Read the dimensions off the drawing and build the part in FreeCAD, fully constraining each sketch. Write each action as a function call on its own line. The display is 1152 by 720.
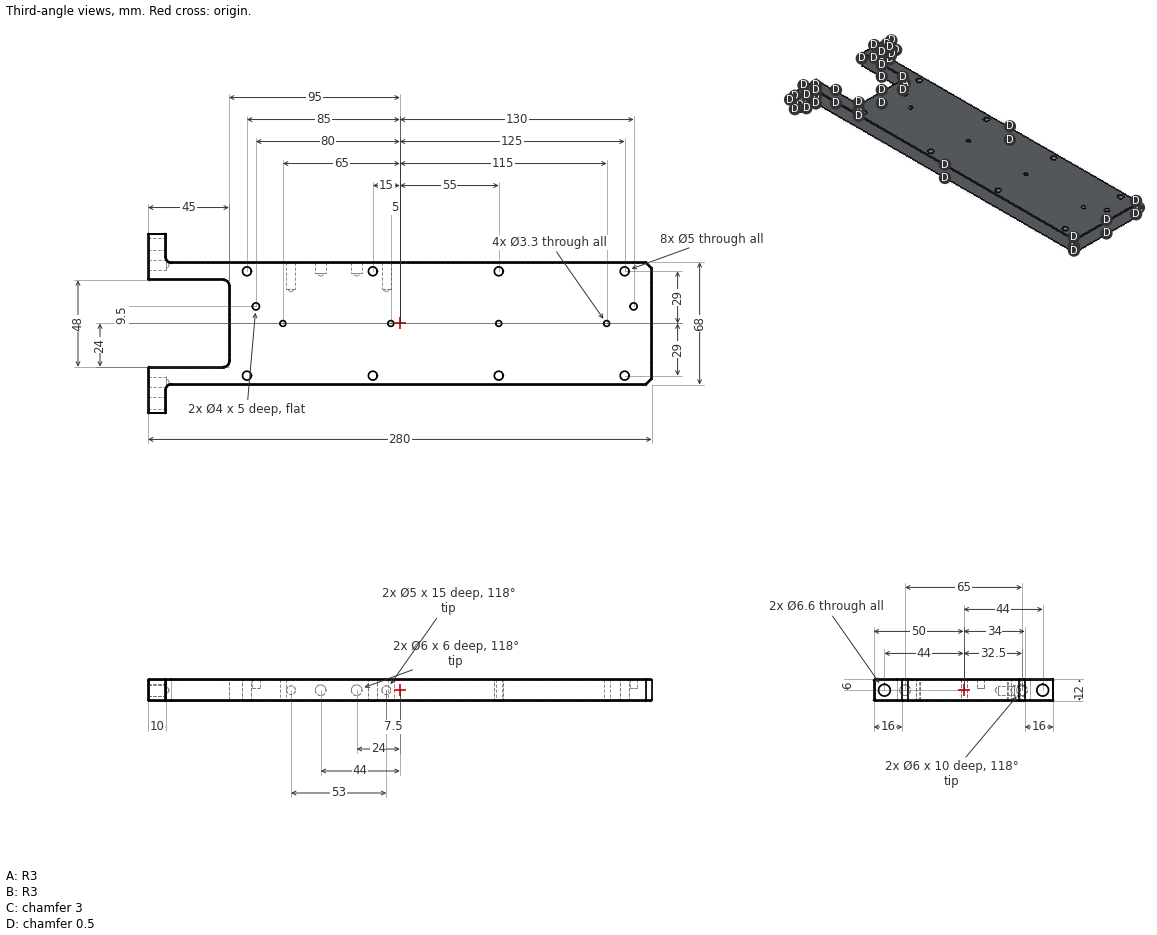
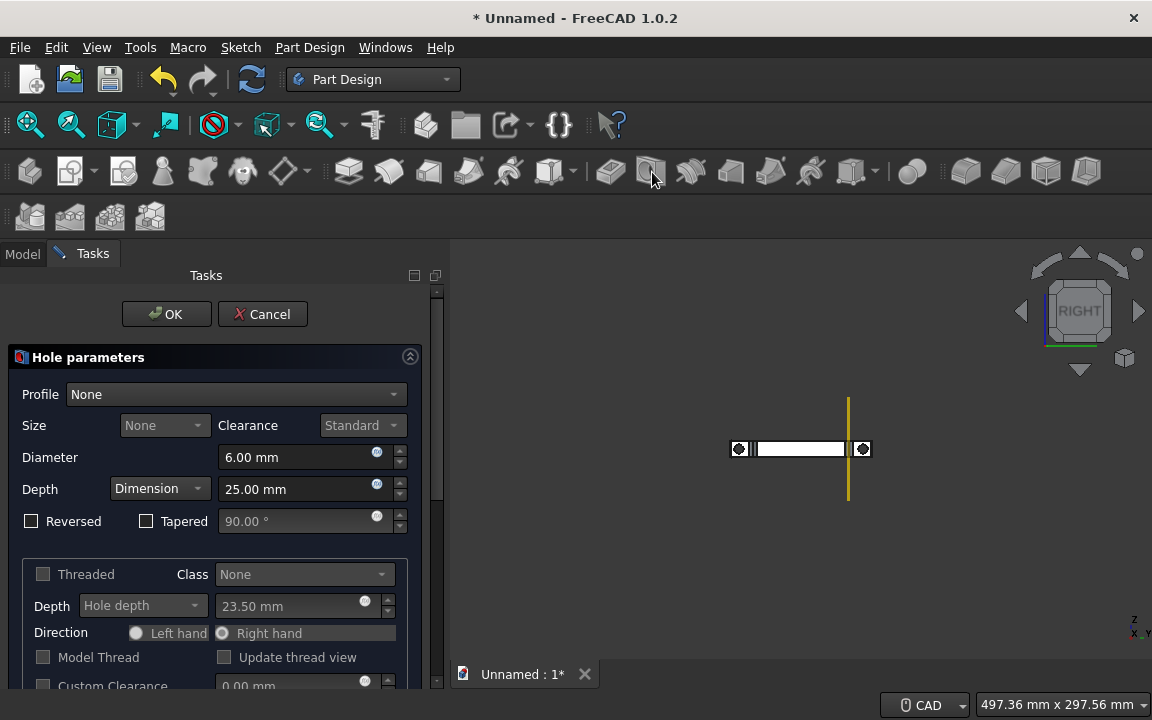
triple_click(305, 457)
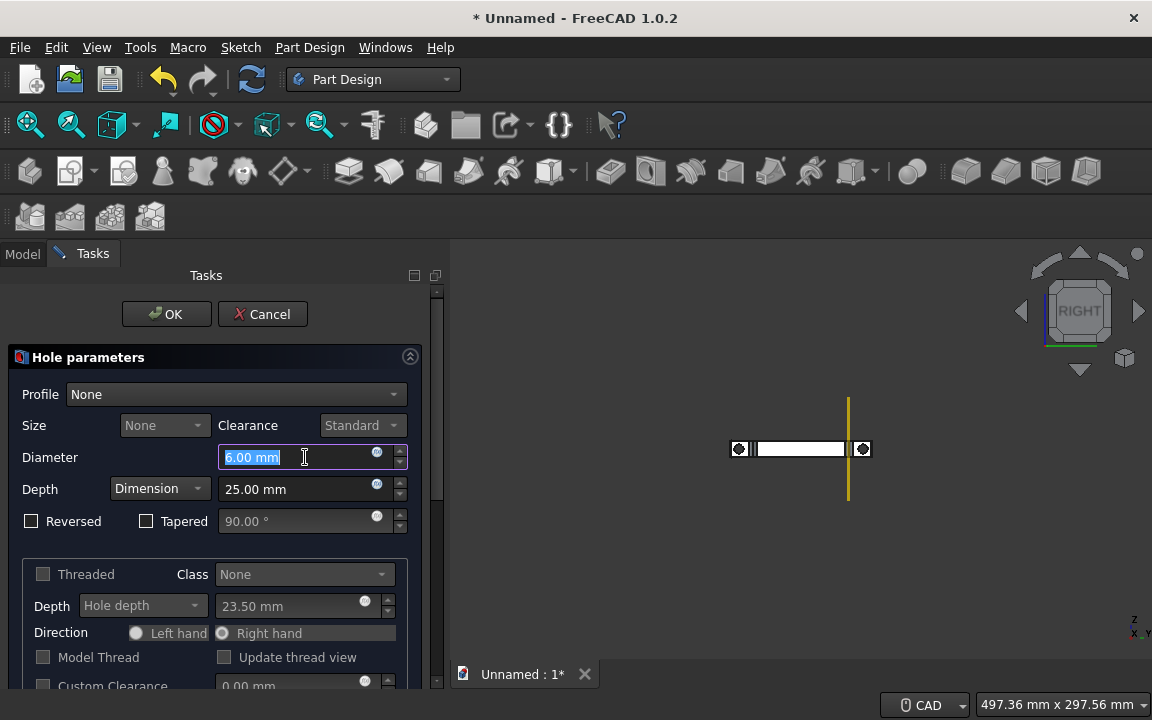
text(5)
key(Tab)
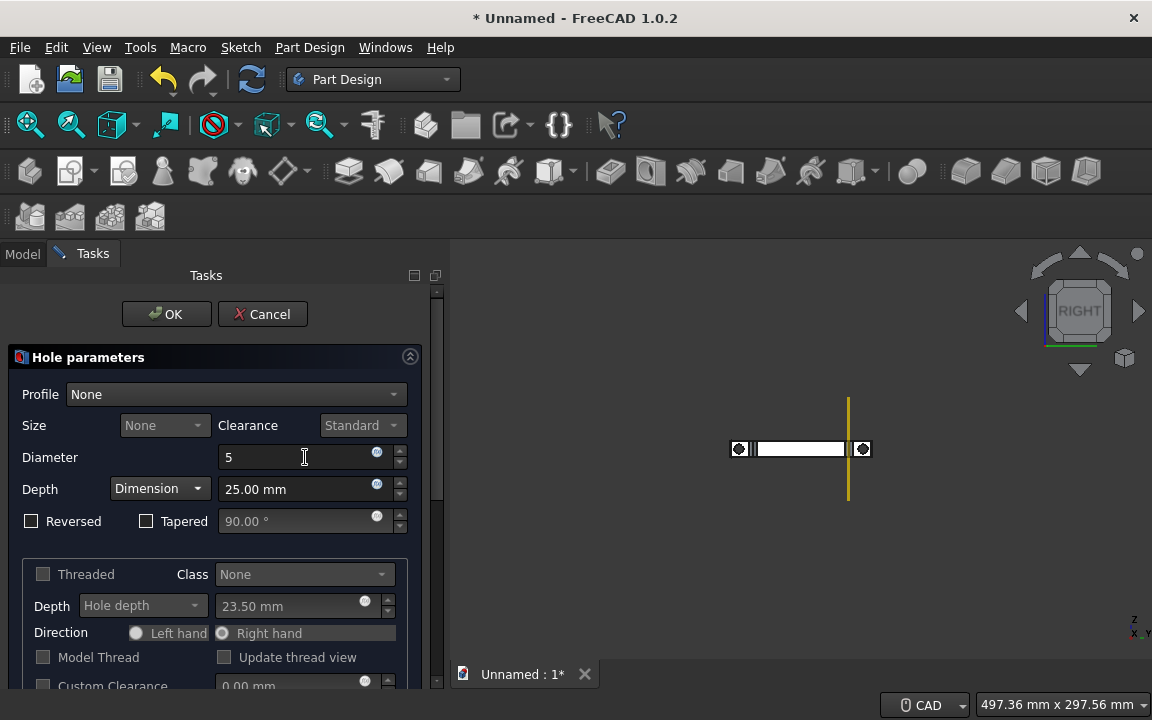
triple_click(305, 489)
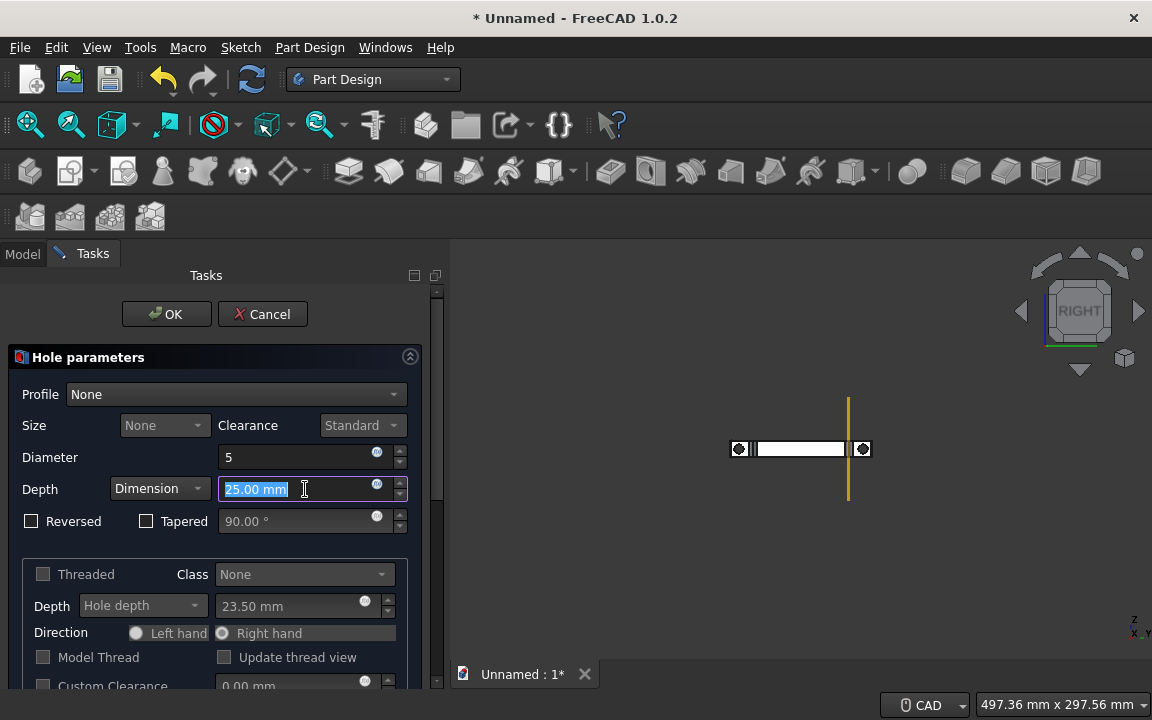
text(15)
key(Tab)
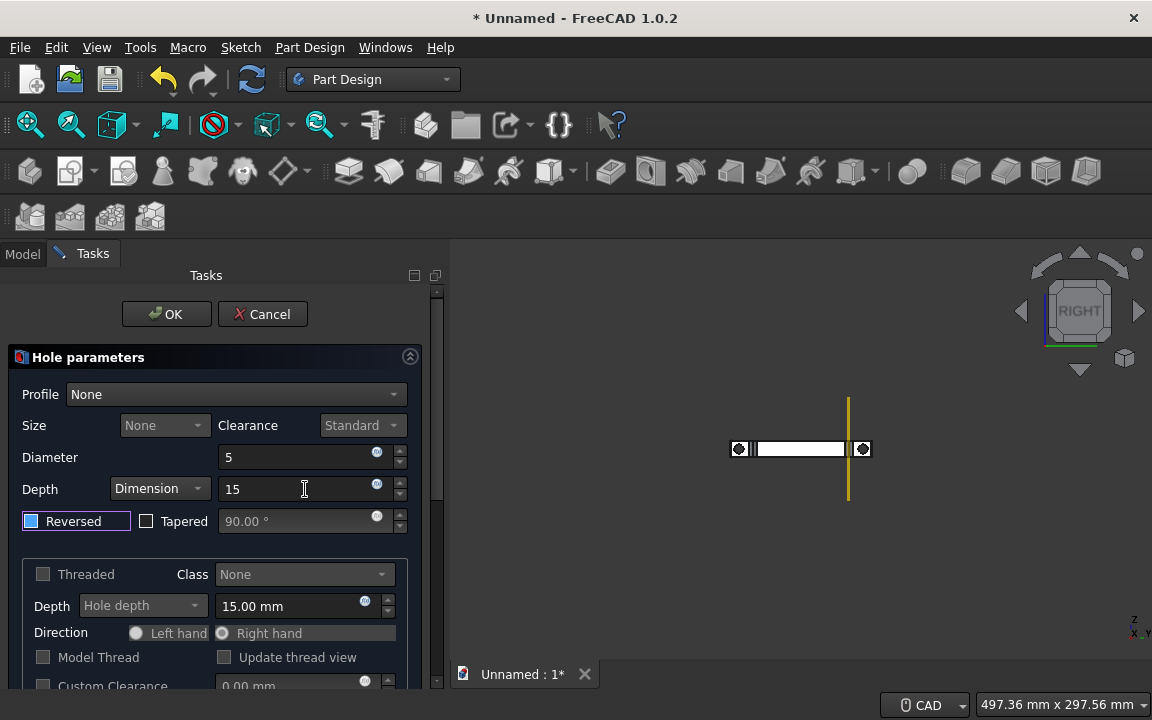
click(30, 521)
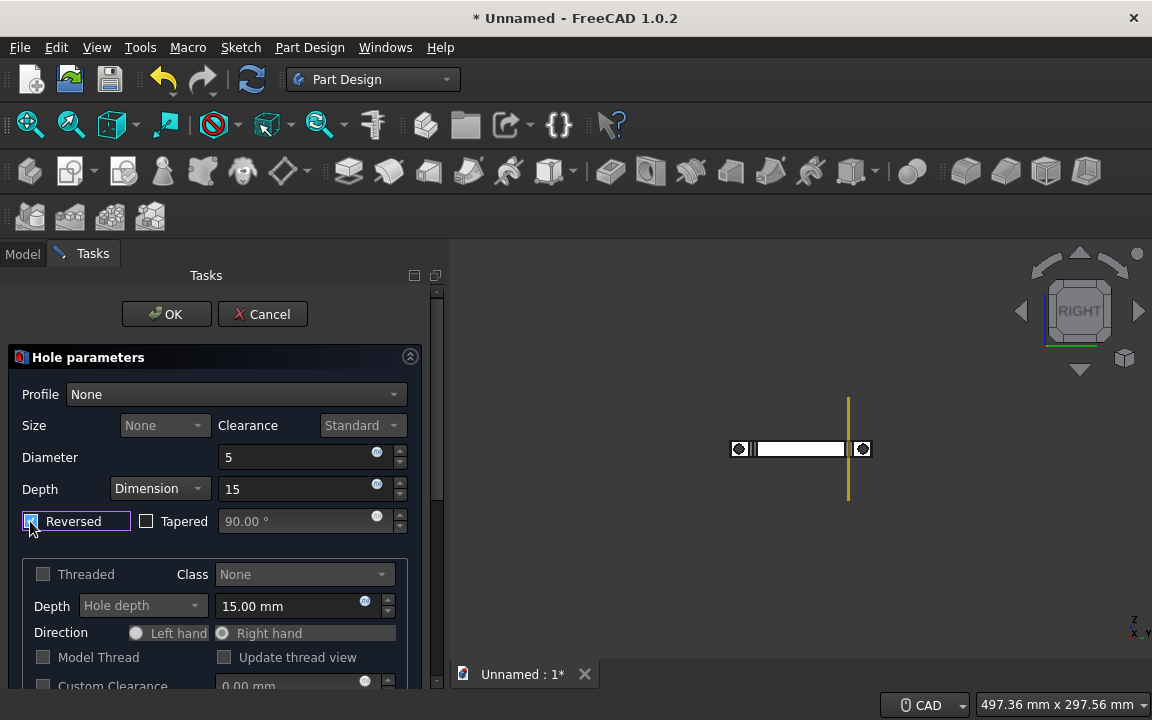
click(167, 314)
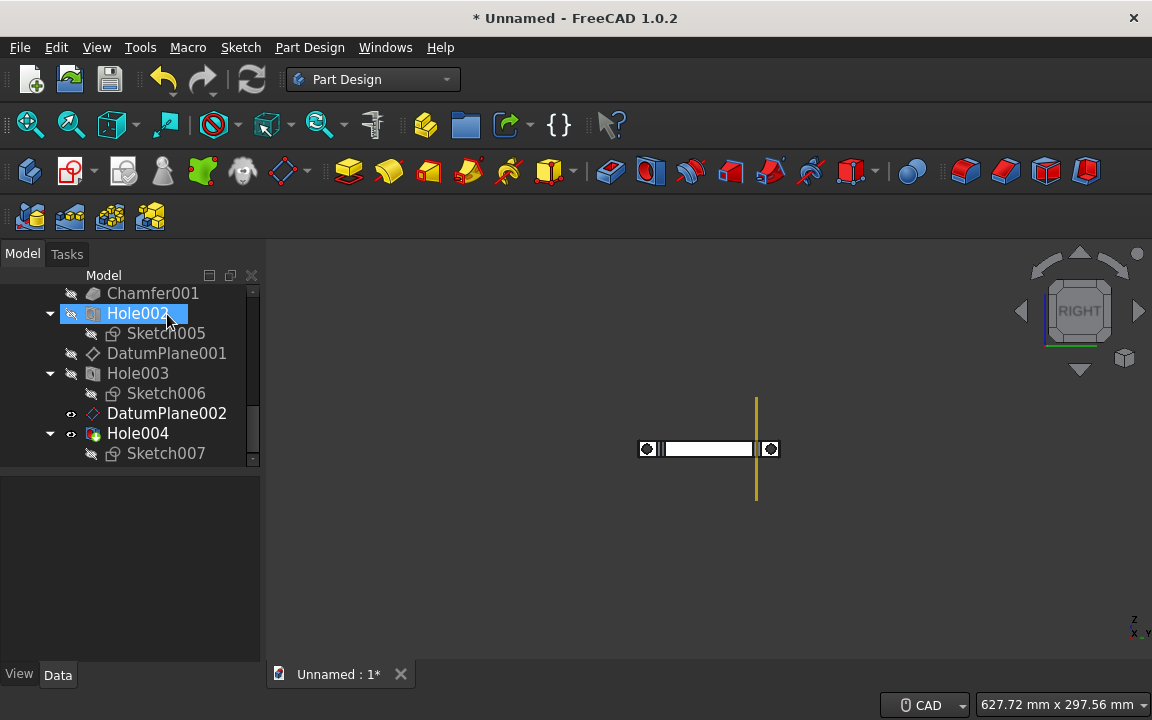
click(116, 414)
key(space)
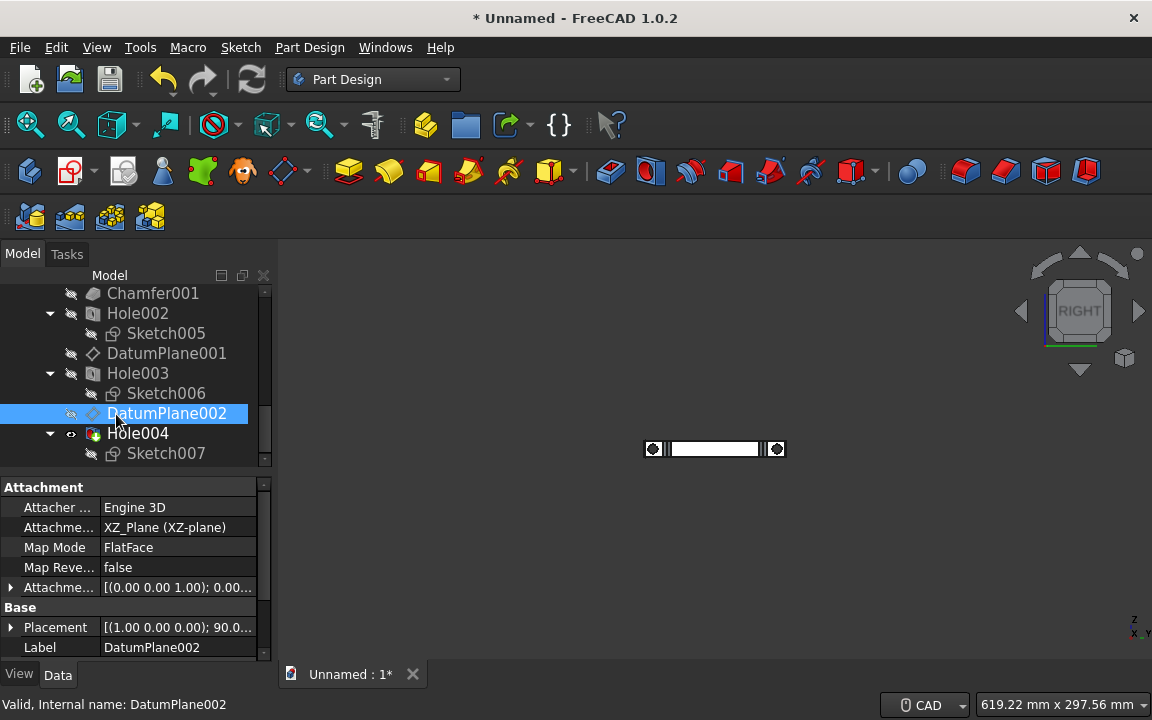
key(v)
key(f)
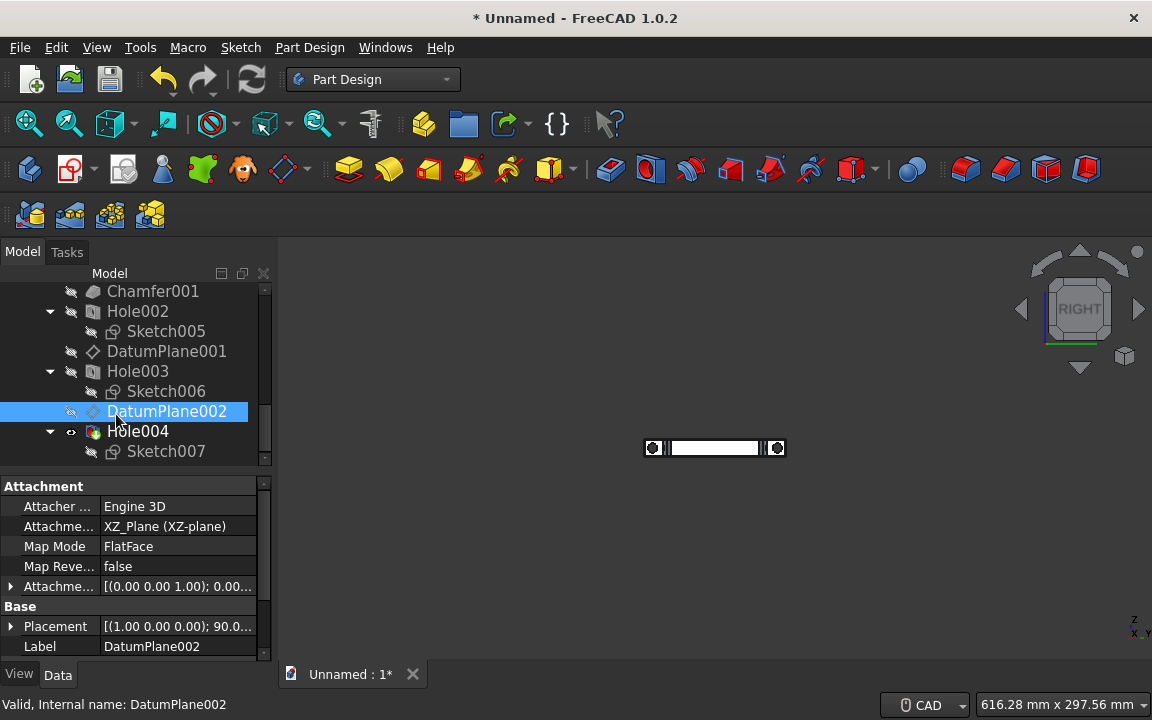
key(0)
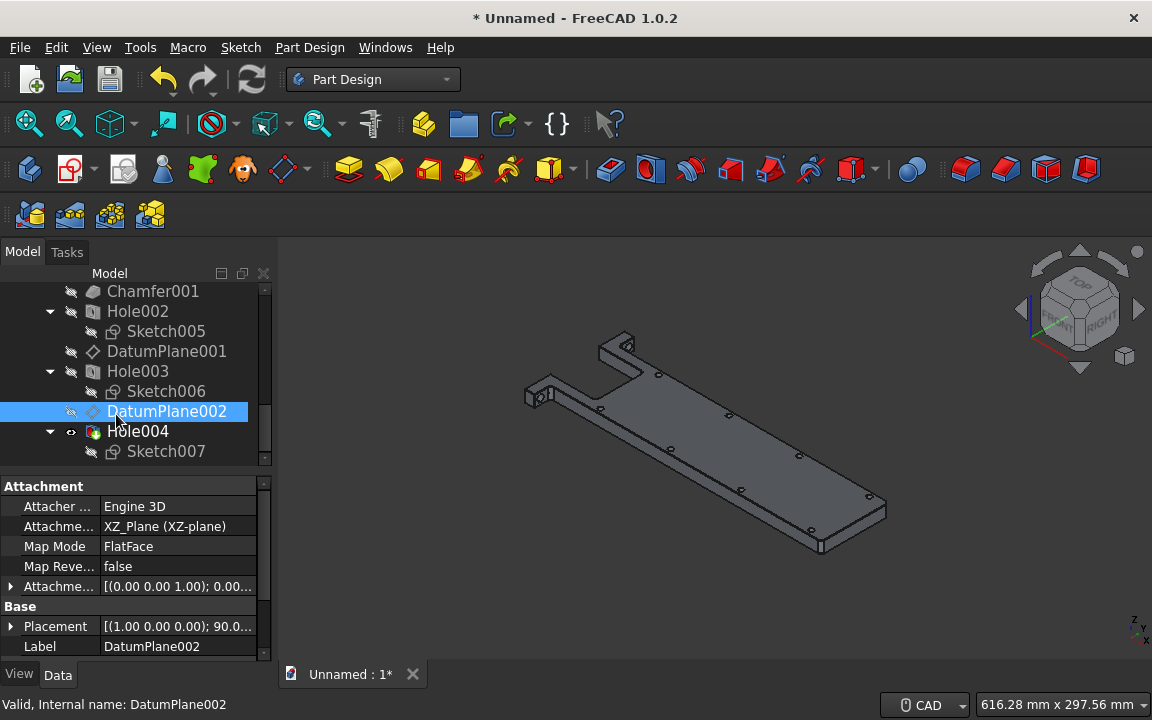
click(795, 486)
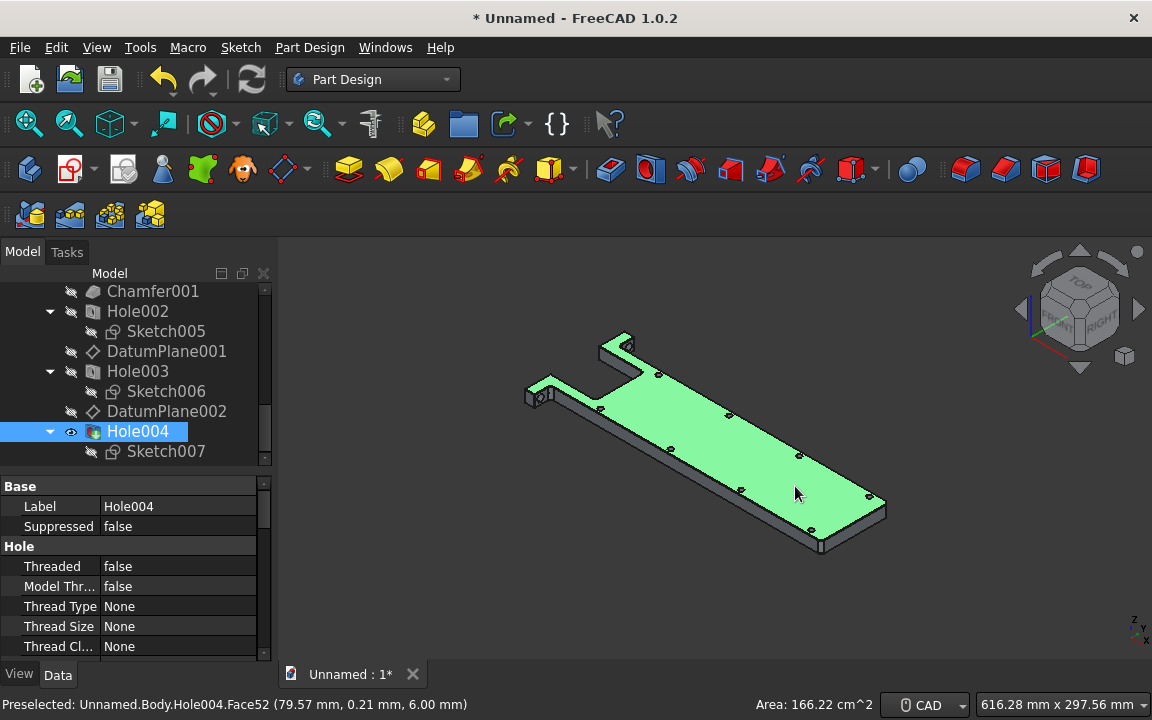
click(70, 170)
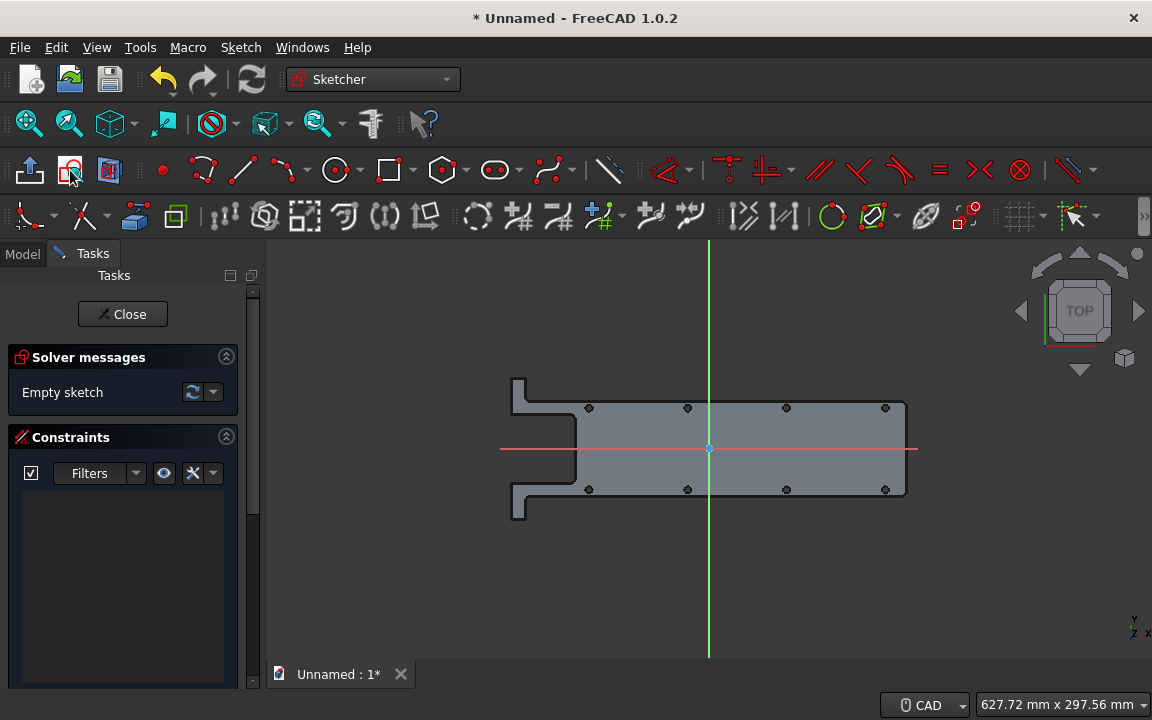
scroll(871, 449, up, 3)